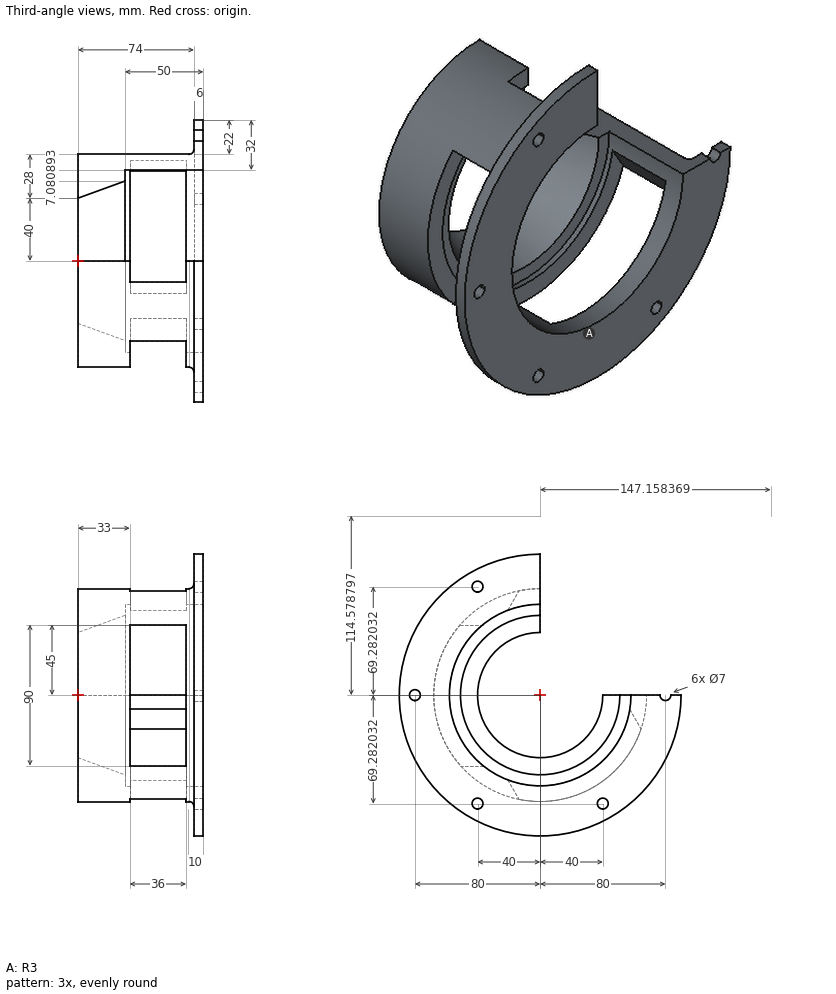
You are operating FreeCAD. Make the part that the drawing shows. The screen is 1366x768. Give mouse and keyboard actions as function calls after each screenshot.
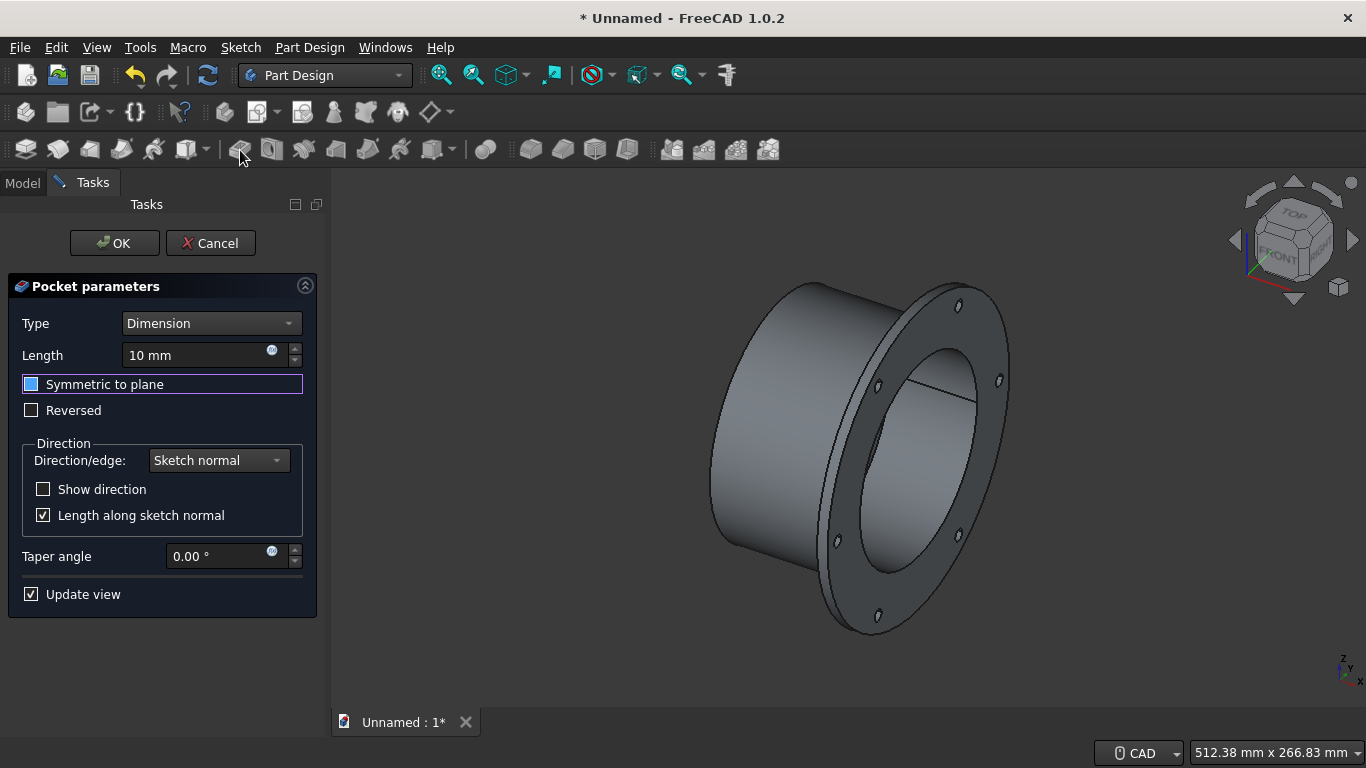
click(115, 243)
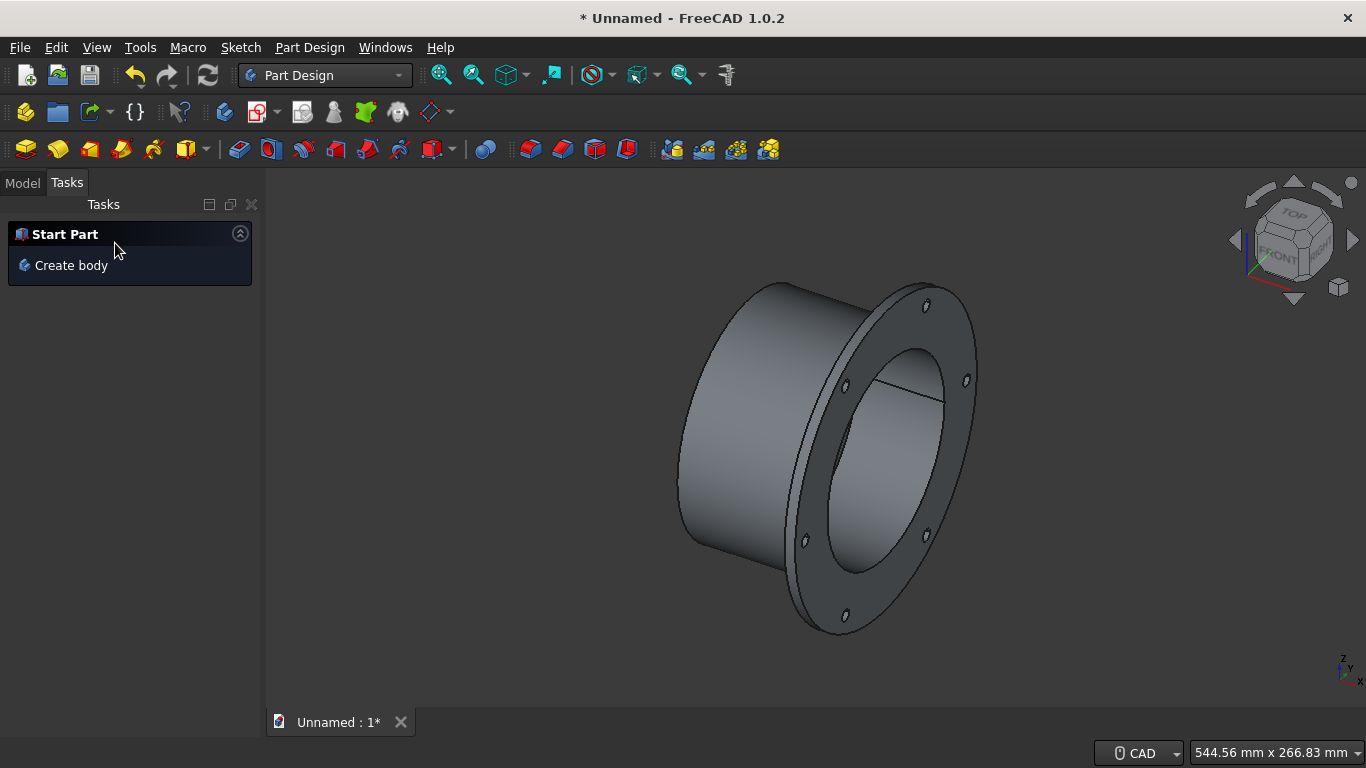
key(0)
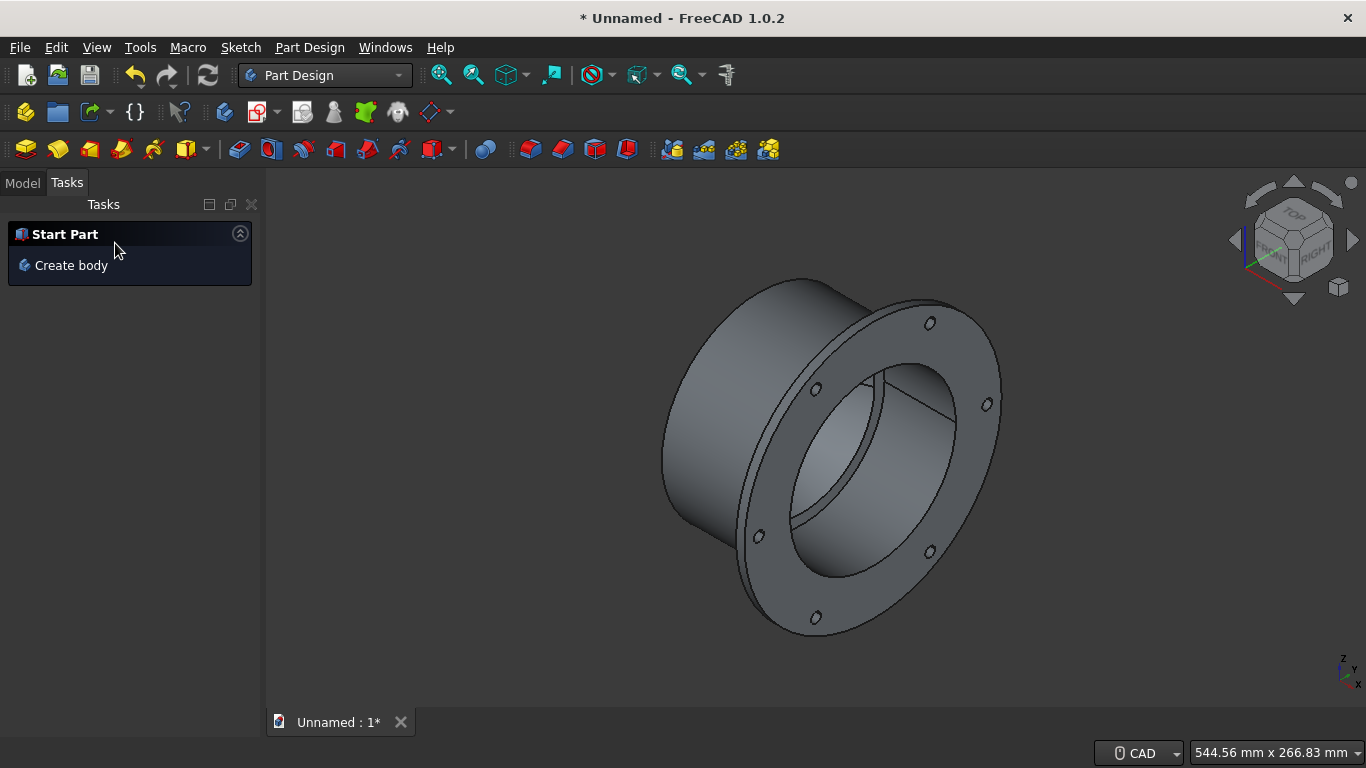
key(2)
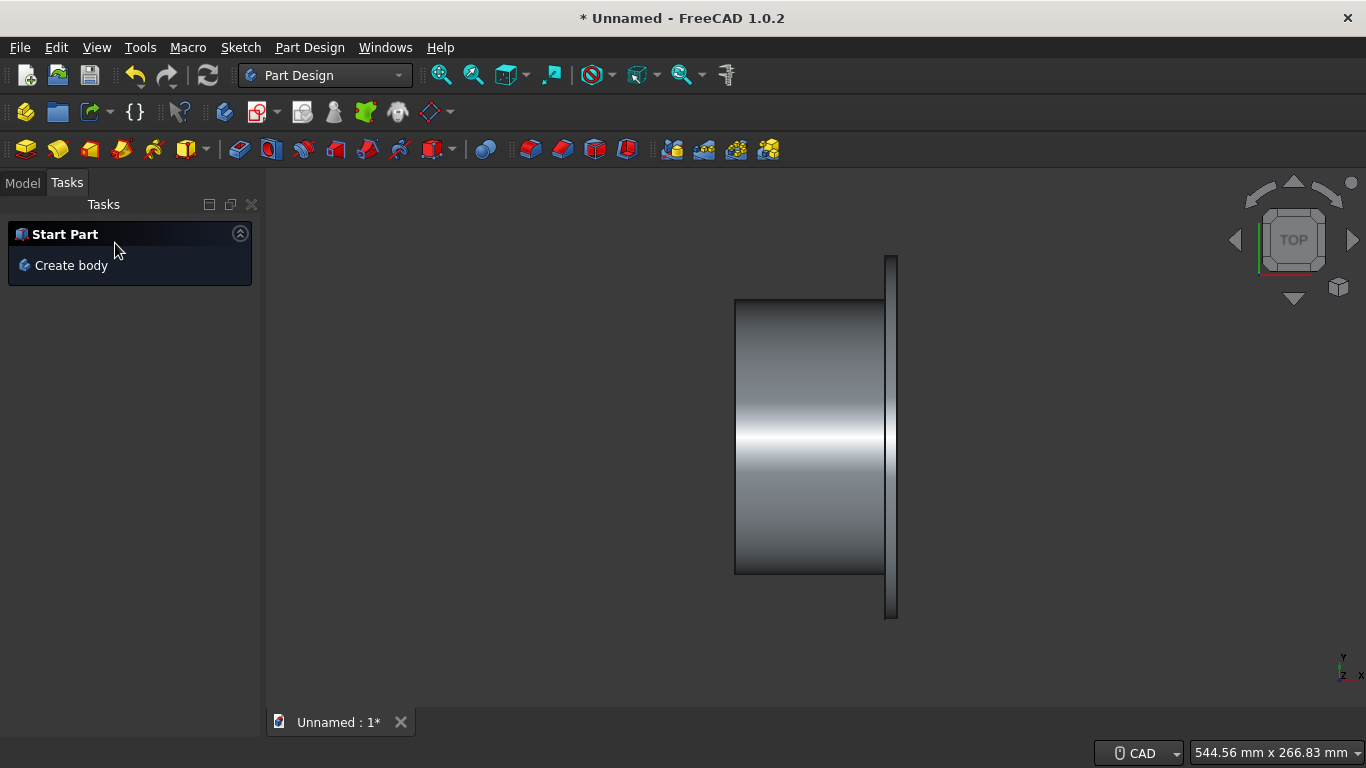
key(1)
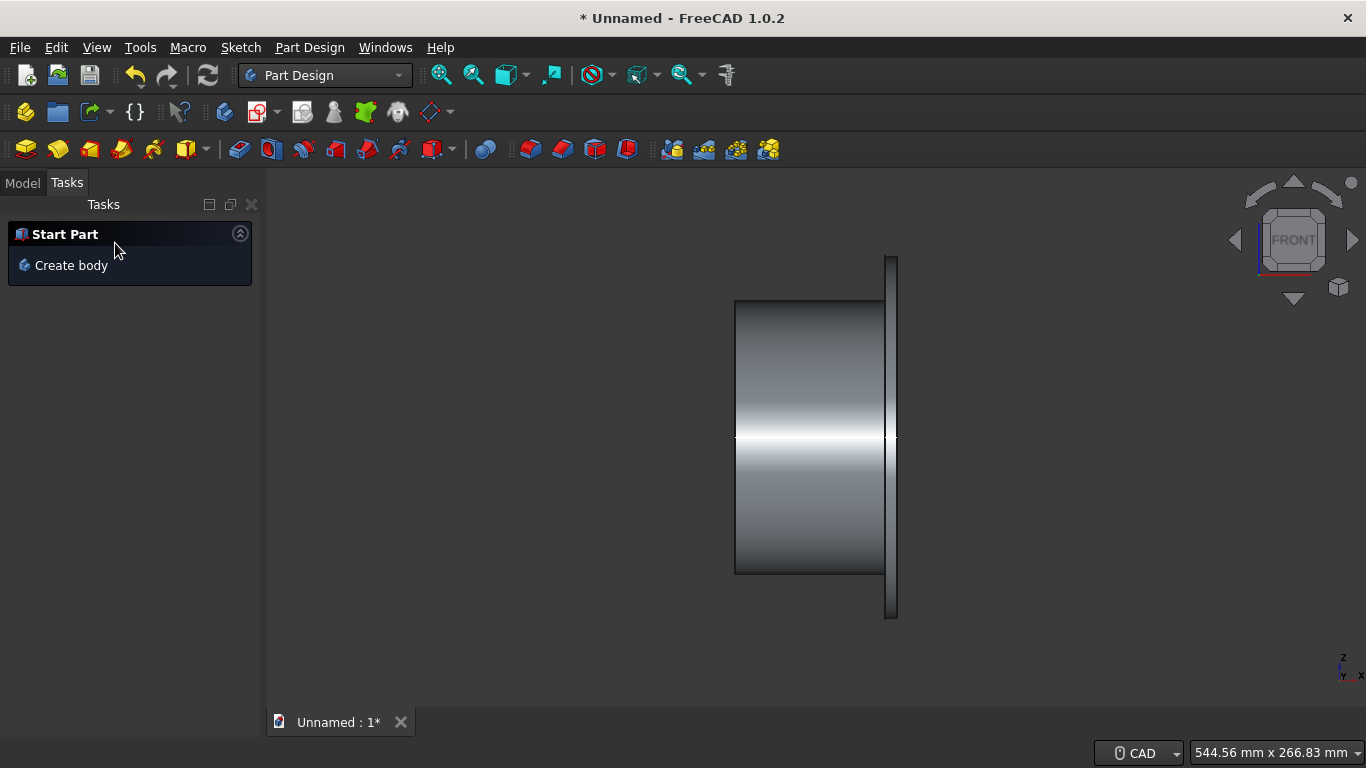
key(3)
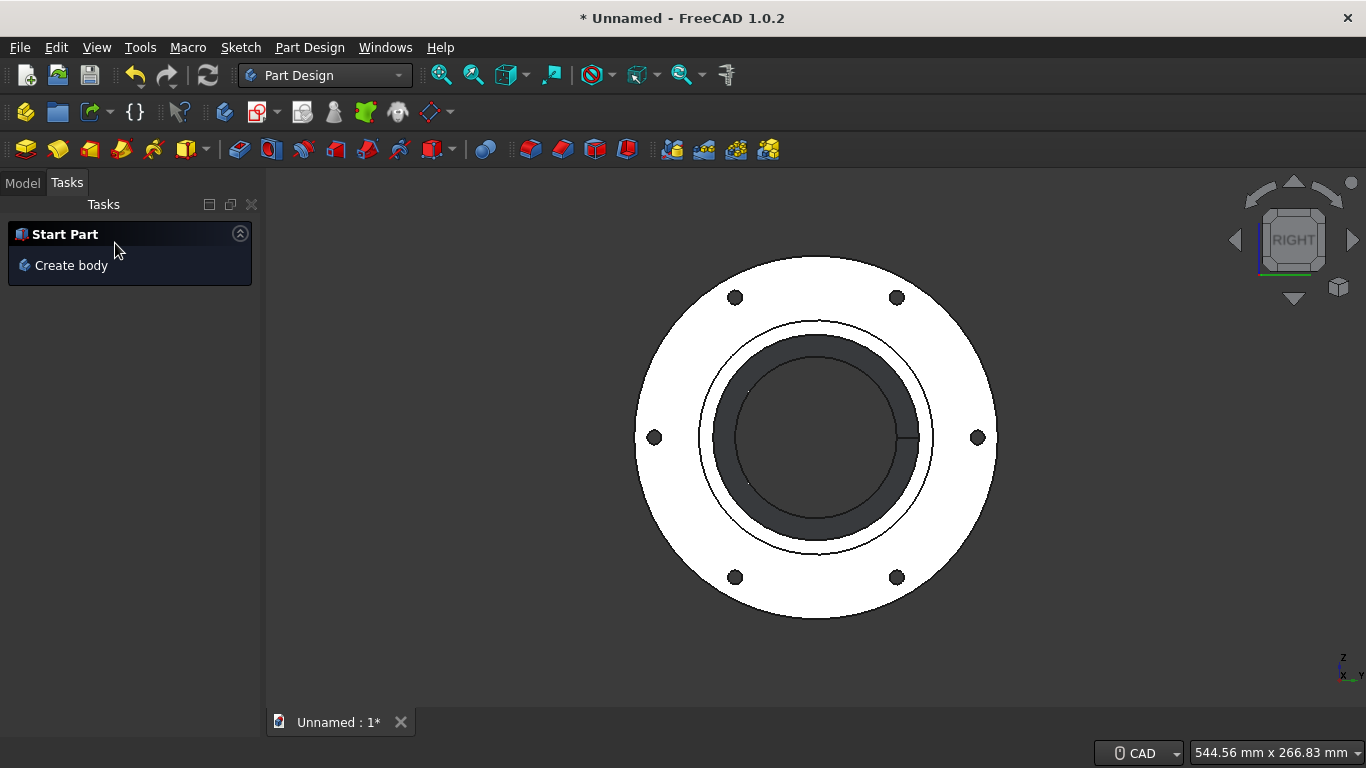
key(5)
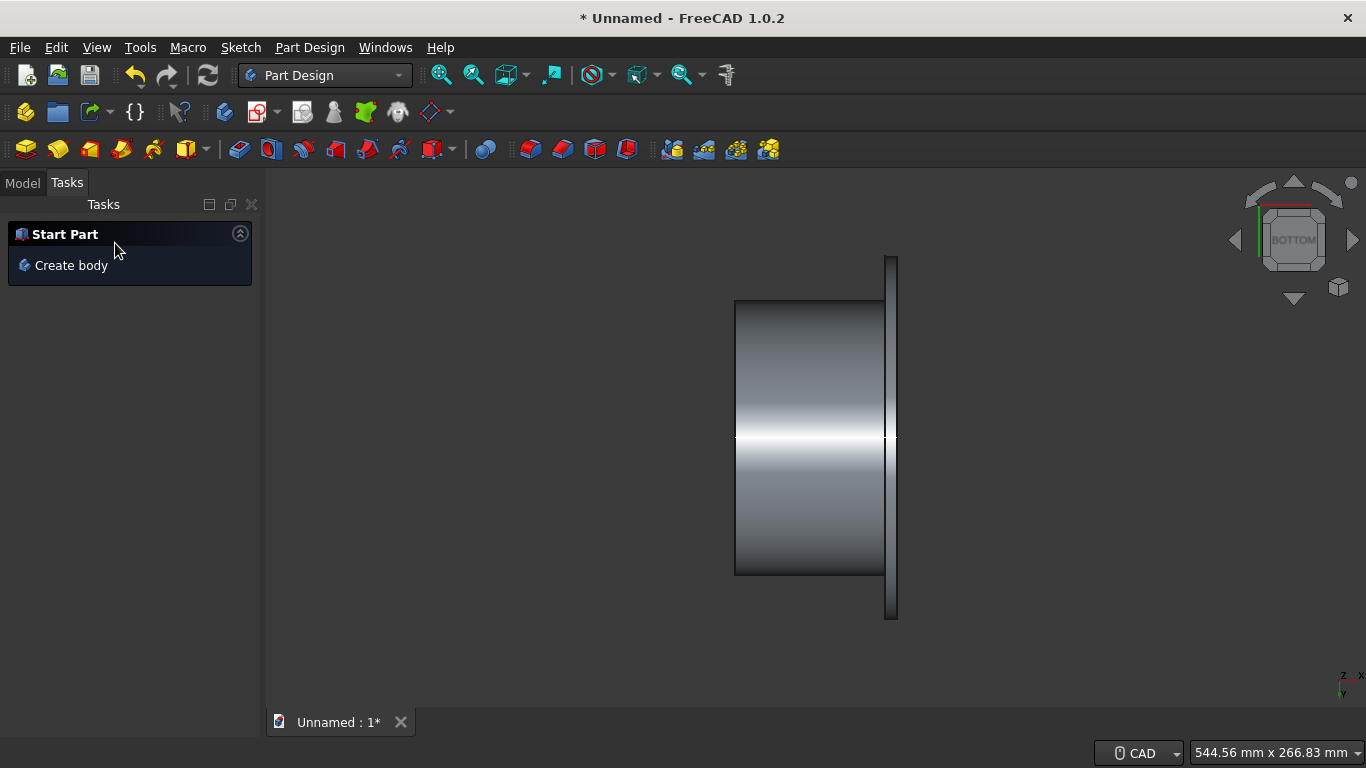
key(4)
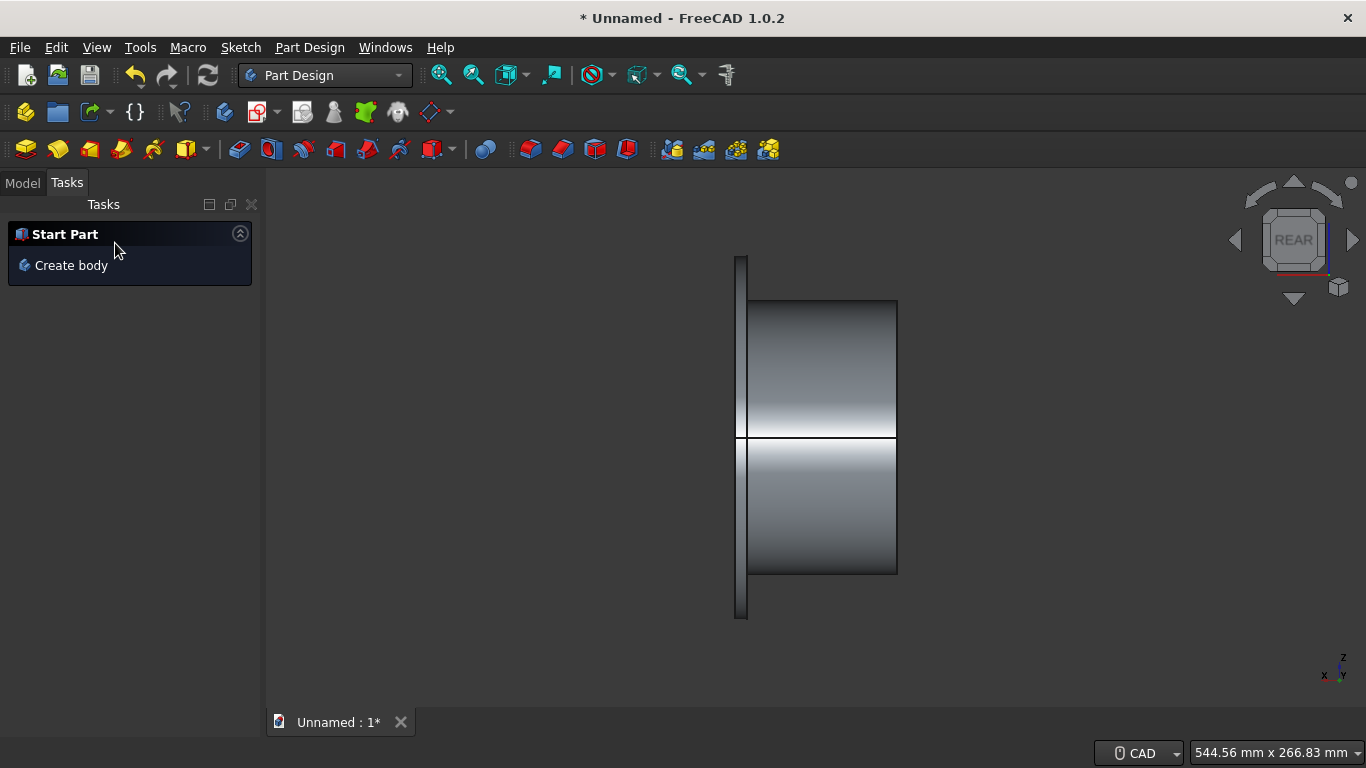
key(6)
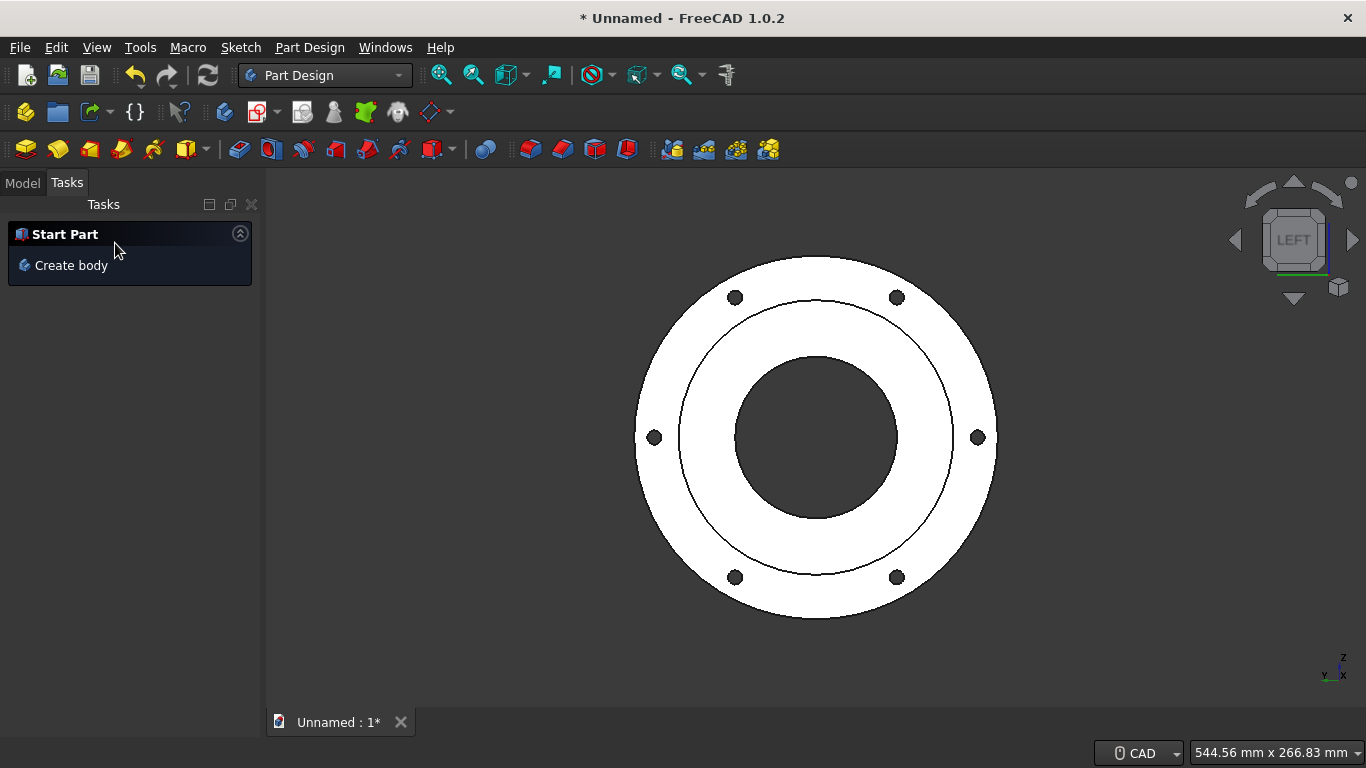
key(v)
key(3)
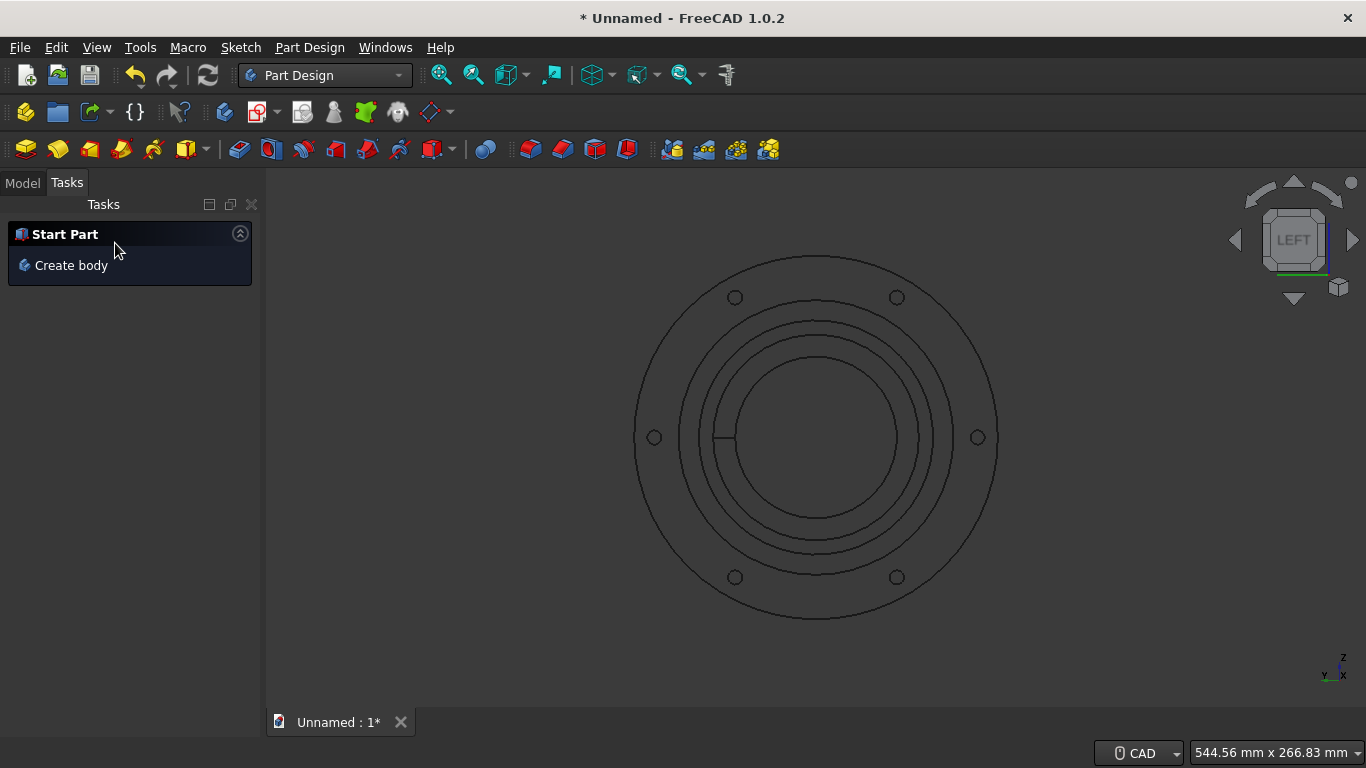
key(0)